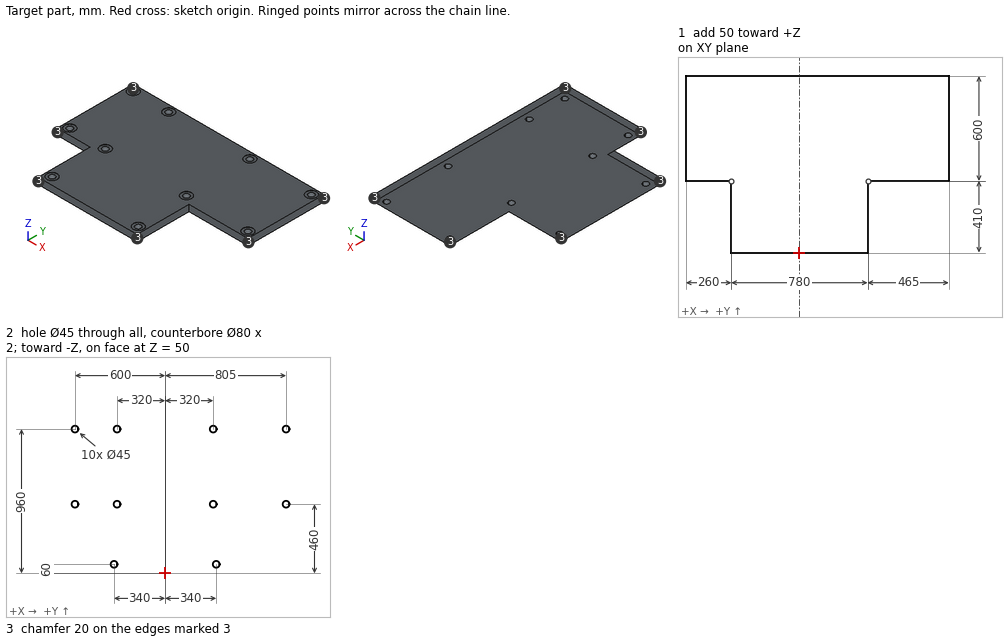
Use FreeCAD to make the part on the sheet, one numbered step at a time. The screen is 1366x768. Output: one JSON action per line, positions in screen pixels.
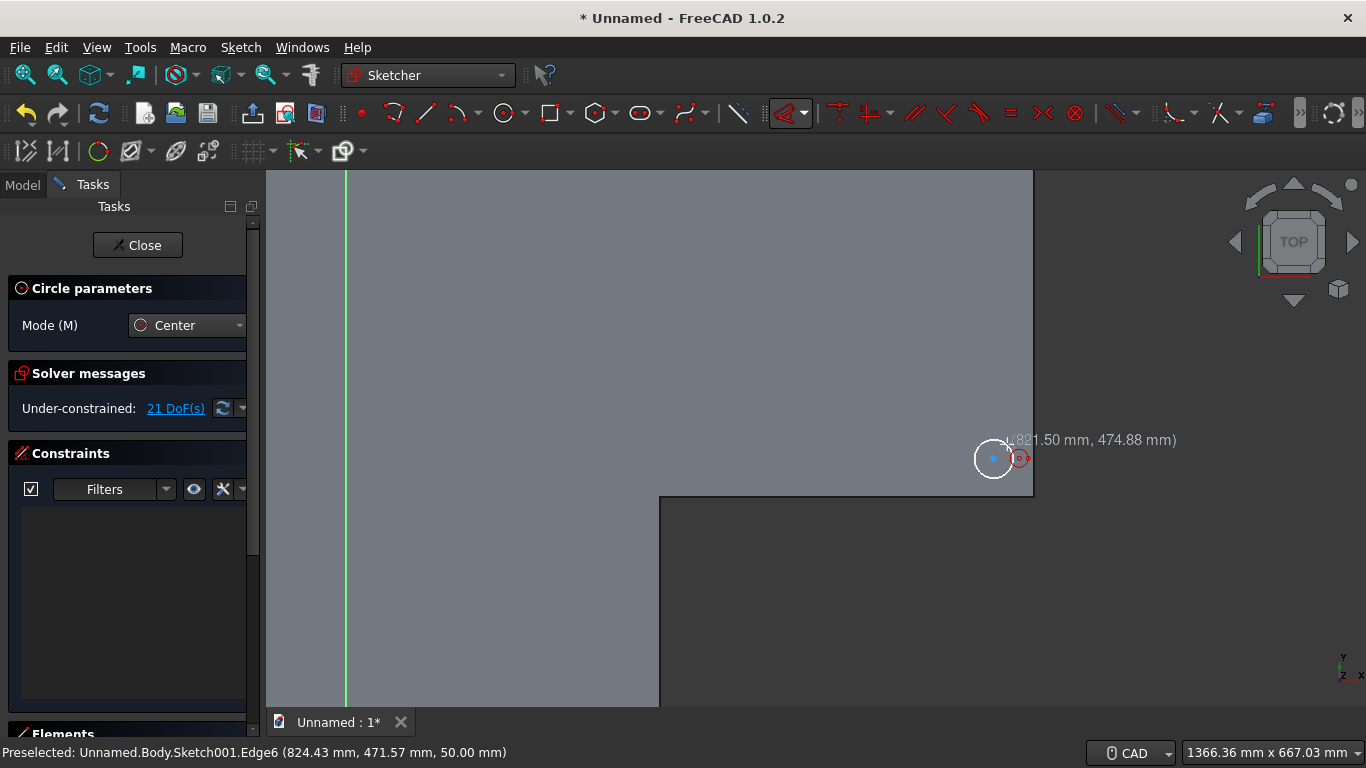
{"action": "scroll", "coordinate": [603, 457], "scroll_direction": "up", "scroll_amount": 2}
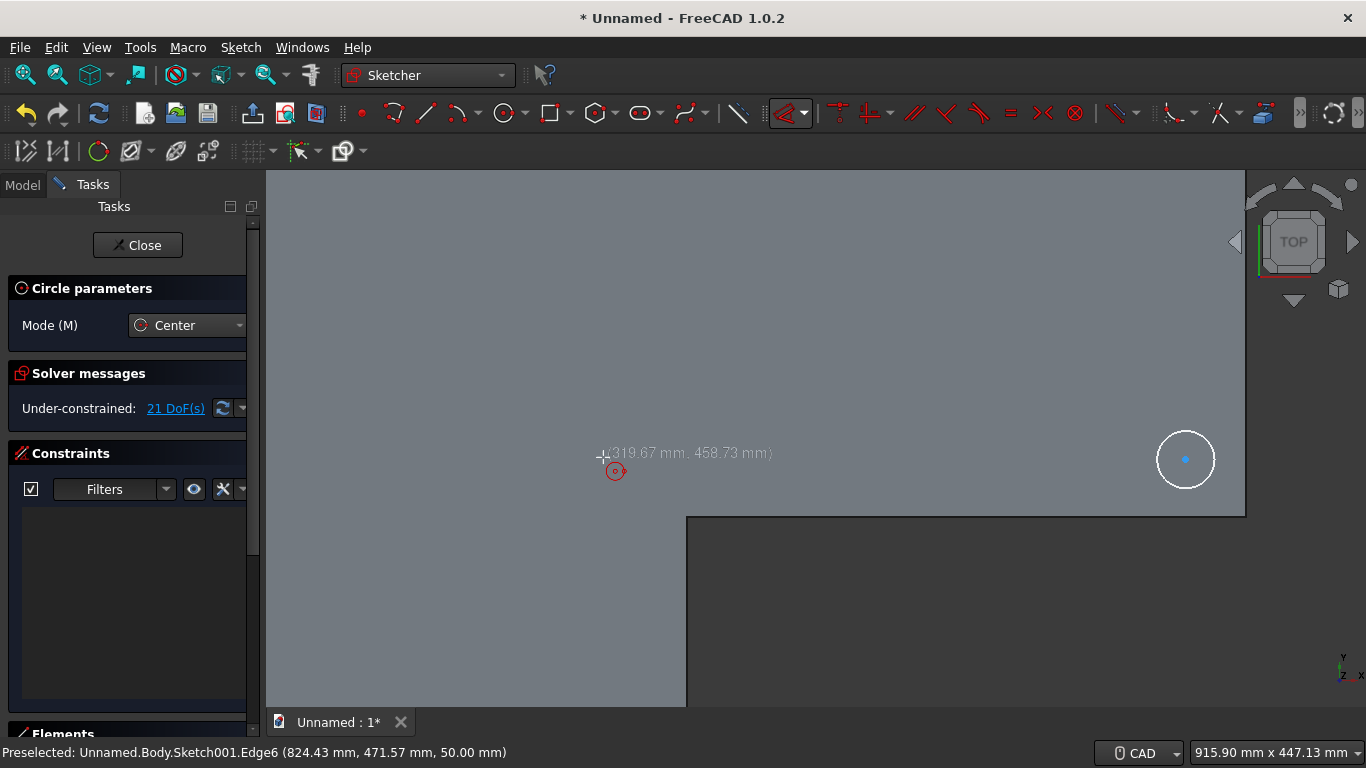
{"action": "scroll", "coordinate": [922, 447], "scroll_direction": "down", "scroll_amount": 6}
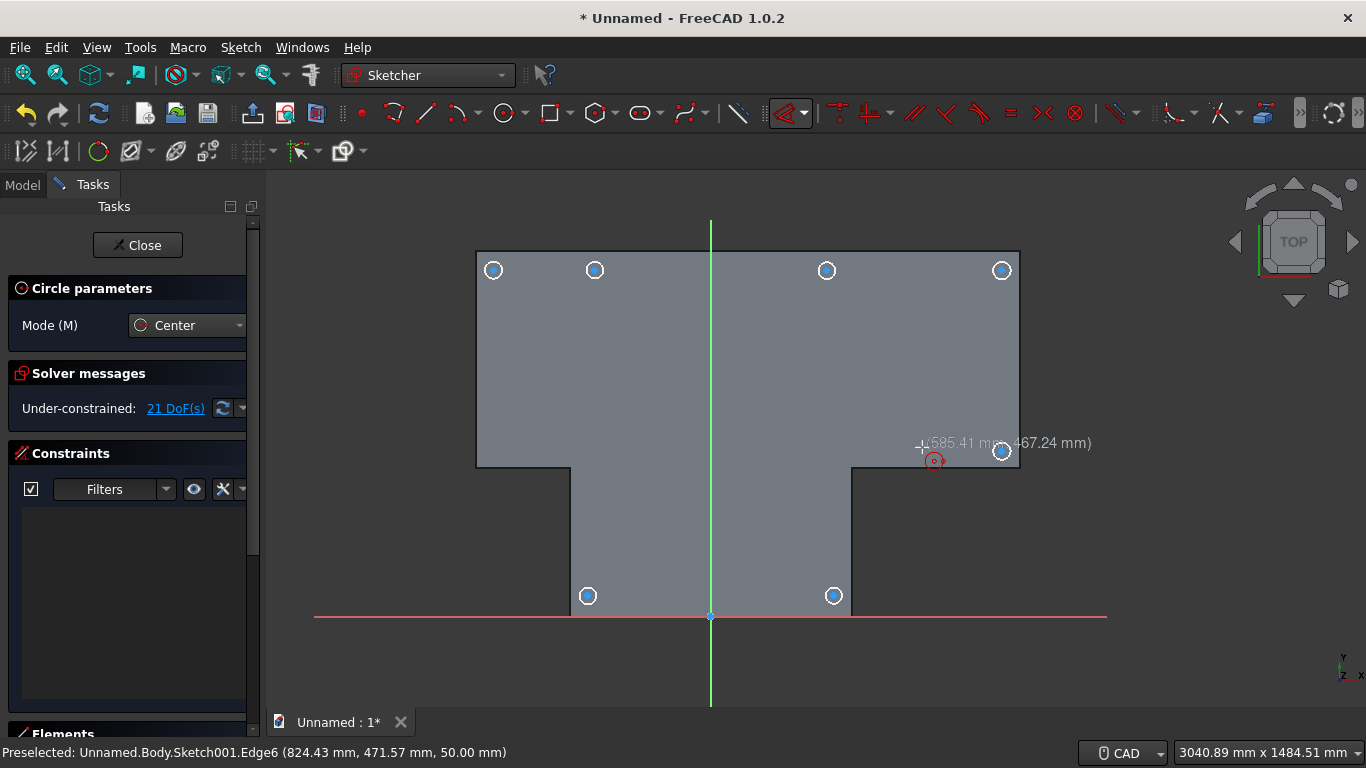
{"action": "left_click", "coordinate": [826, 450]}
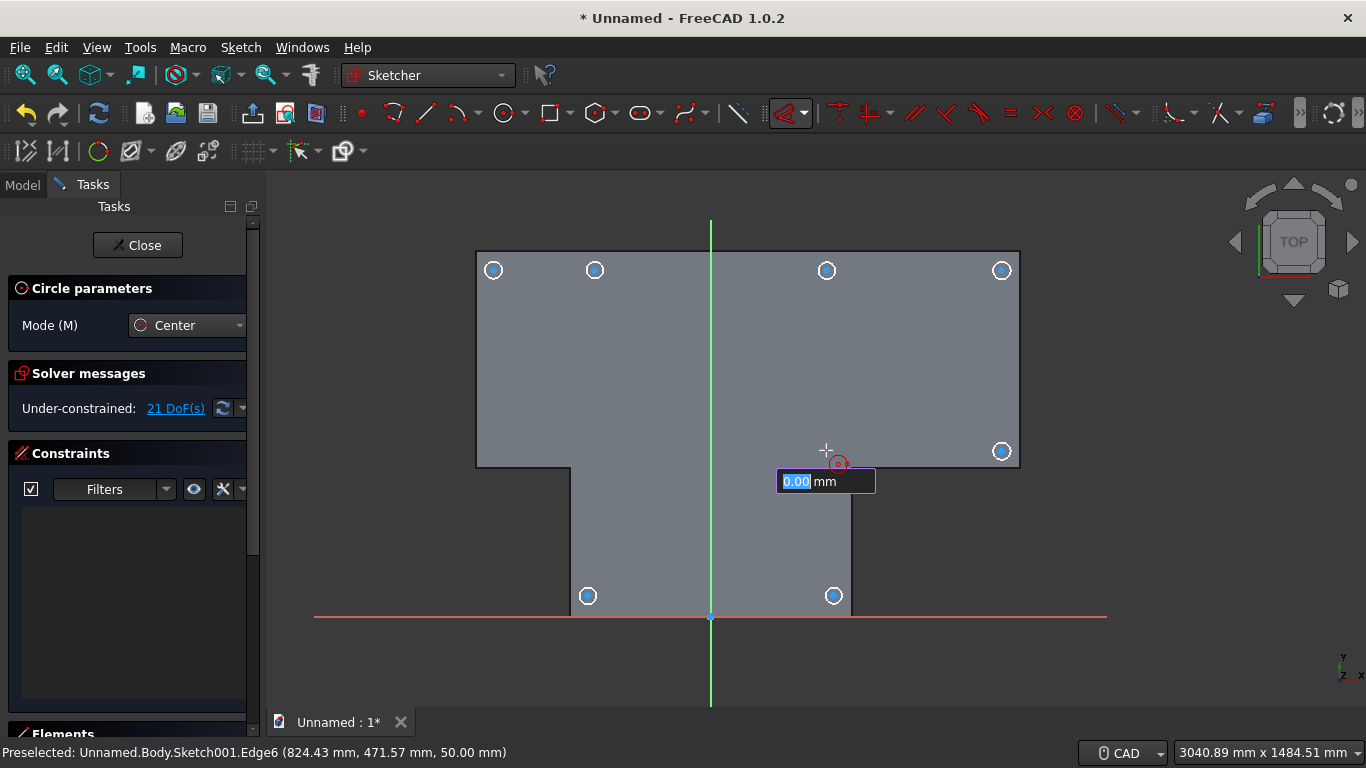
{"action": "scroll", "coordinate": [832, 445], "scroll_direction": "up", "scroll_amount": 4}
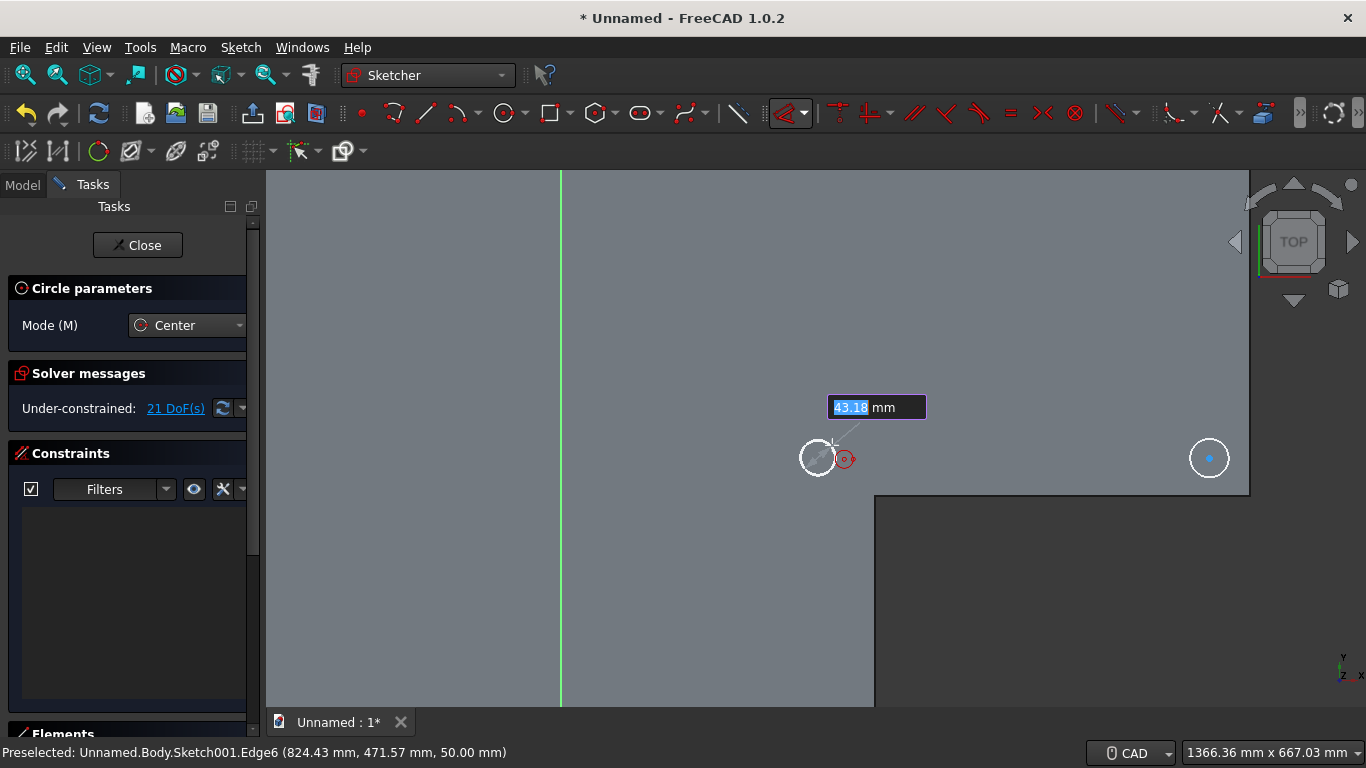
{"action": "left_click", "coordinate": [832, 443]}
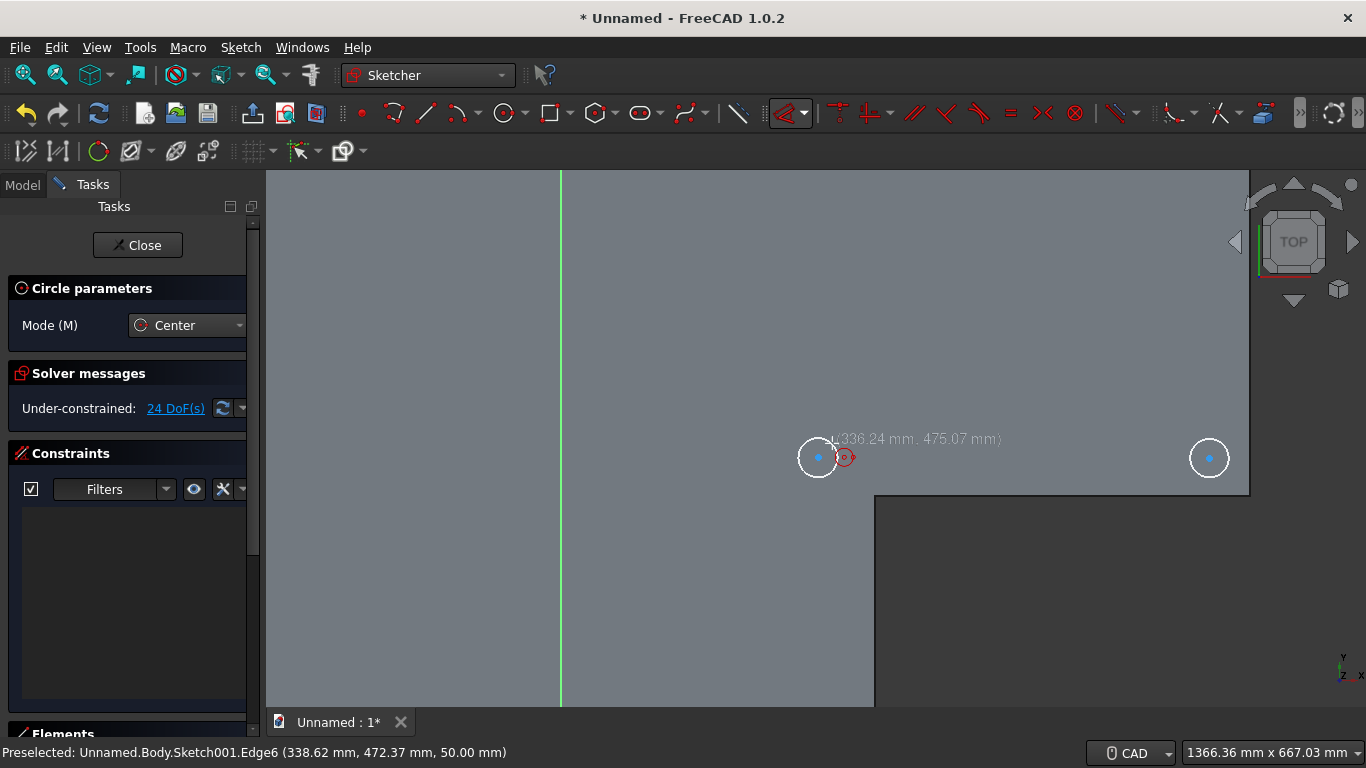
{"action": "scroll", "coordinate": [304, 456], "scroll_direction": "up", "scroll_amount": 2}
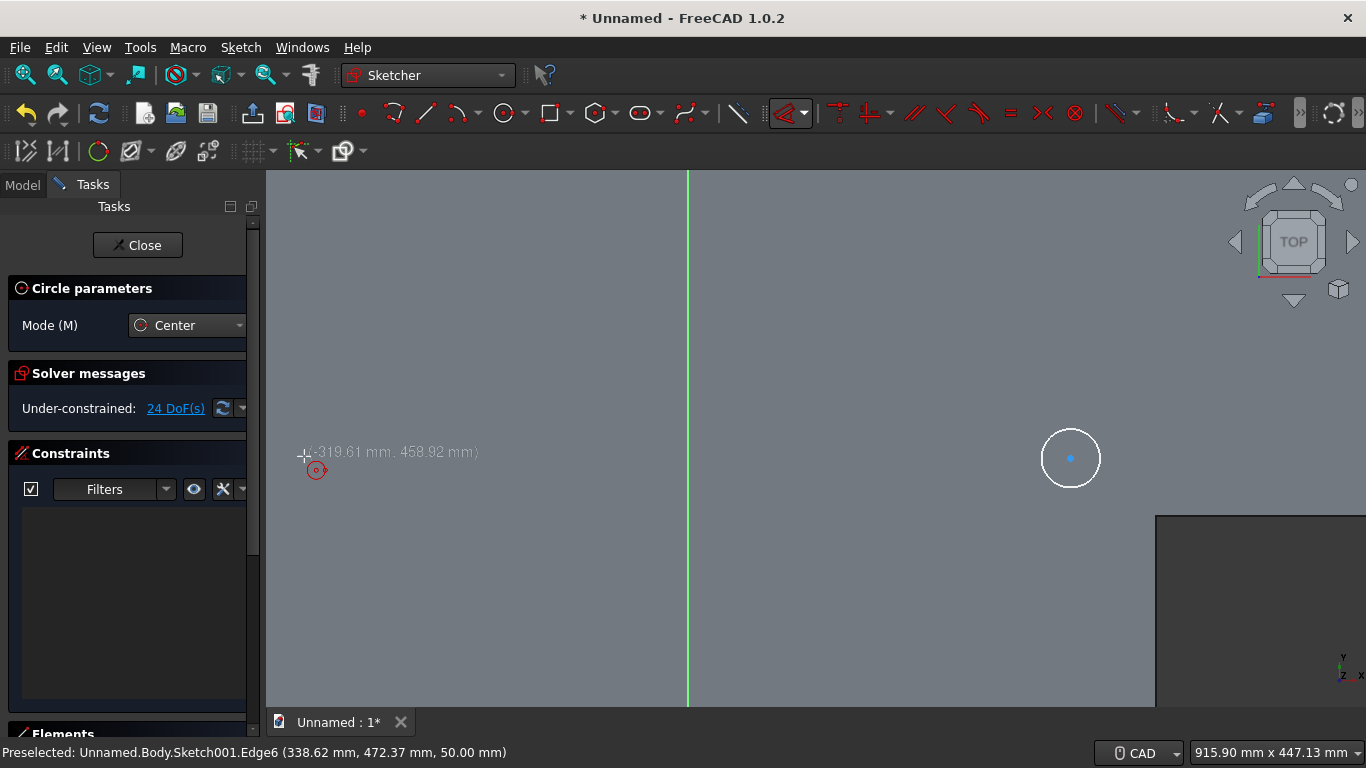
{"action": "scroll", "coordinate": [720, 447], "scroll_direction": "down", "scroll_amount": 6}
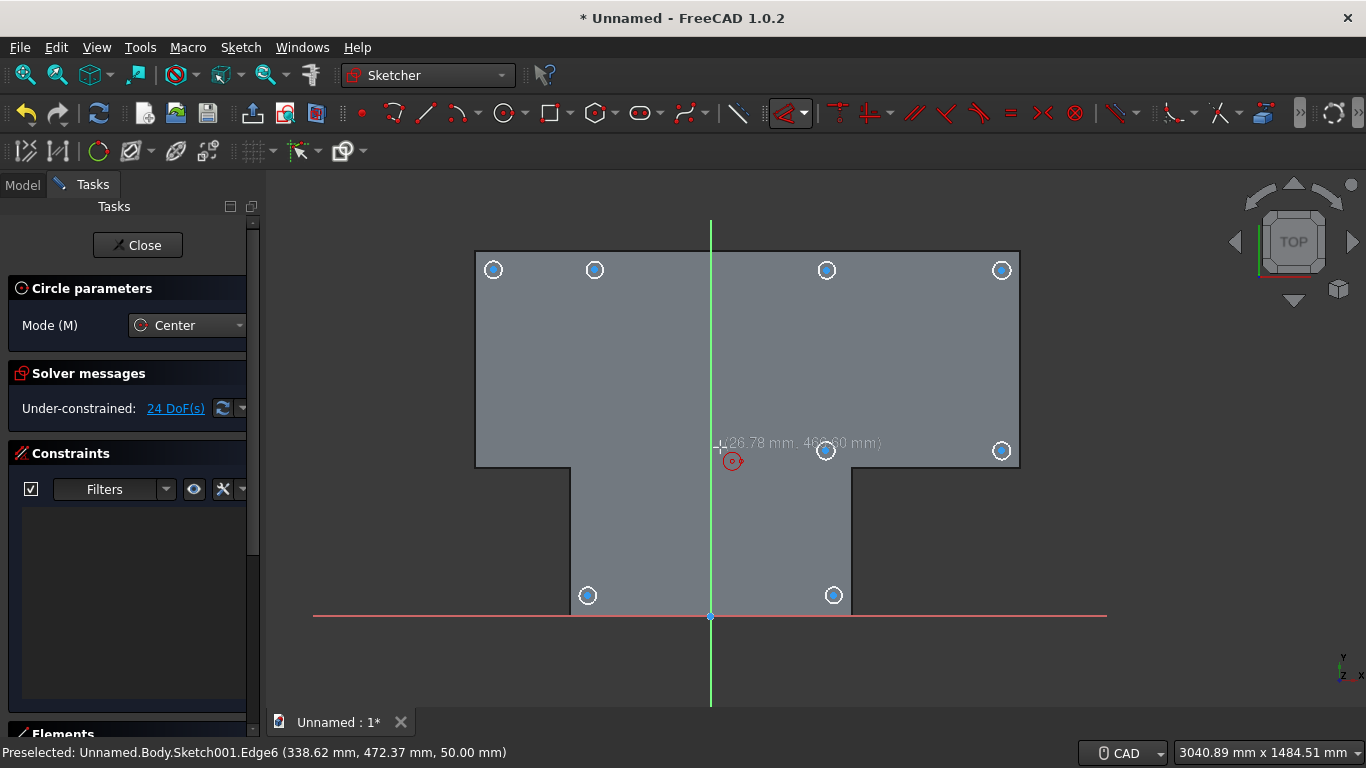
{"action": "left_click", "coordinate": [595, 450]}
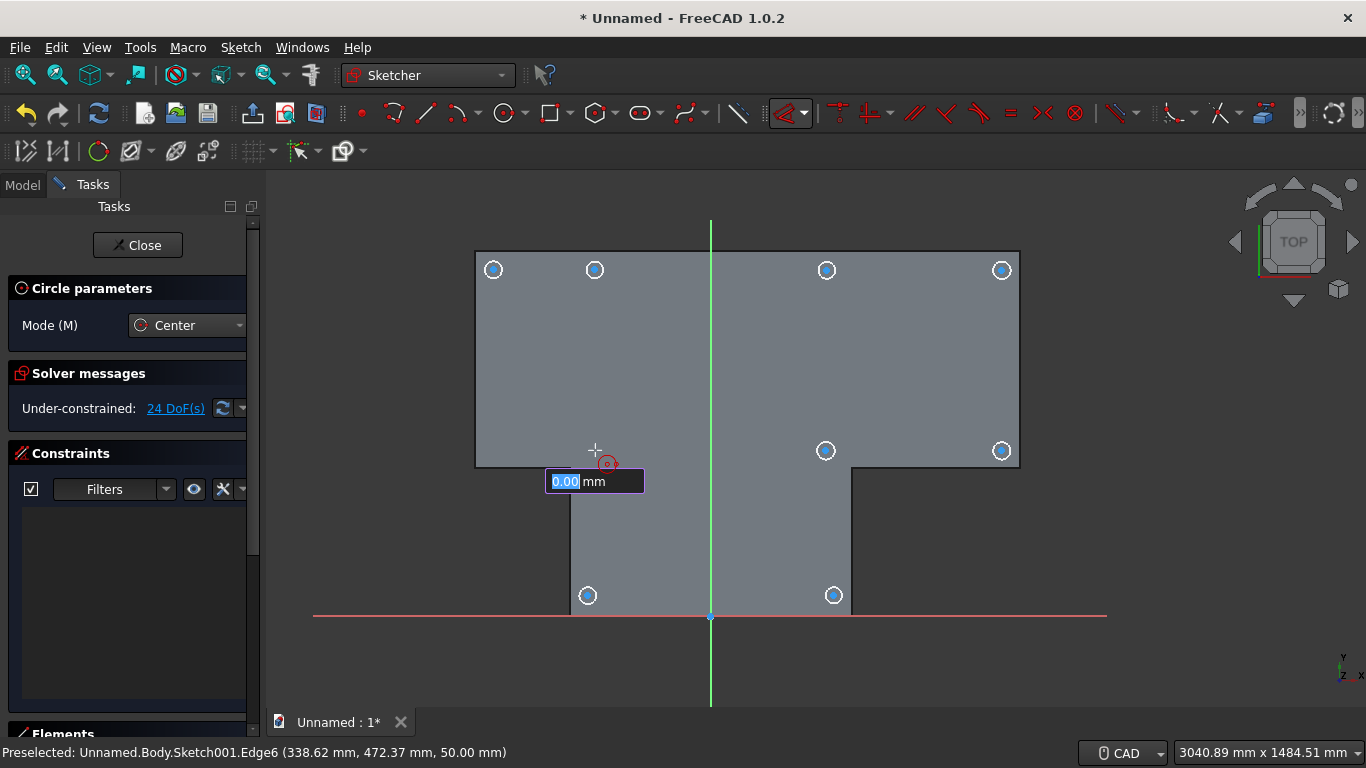
{"action": "scroll", "coordinate": [601, 444], "scroll_direction": "up", "scroll_amount": 4}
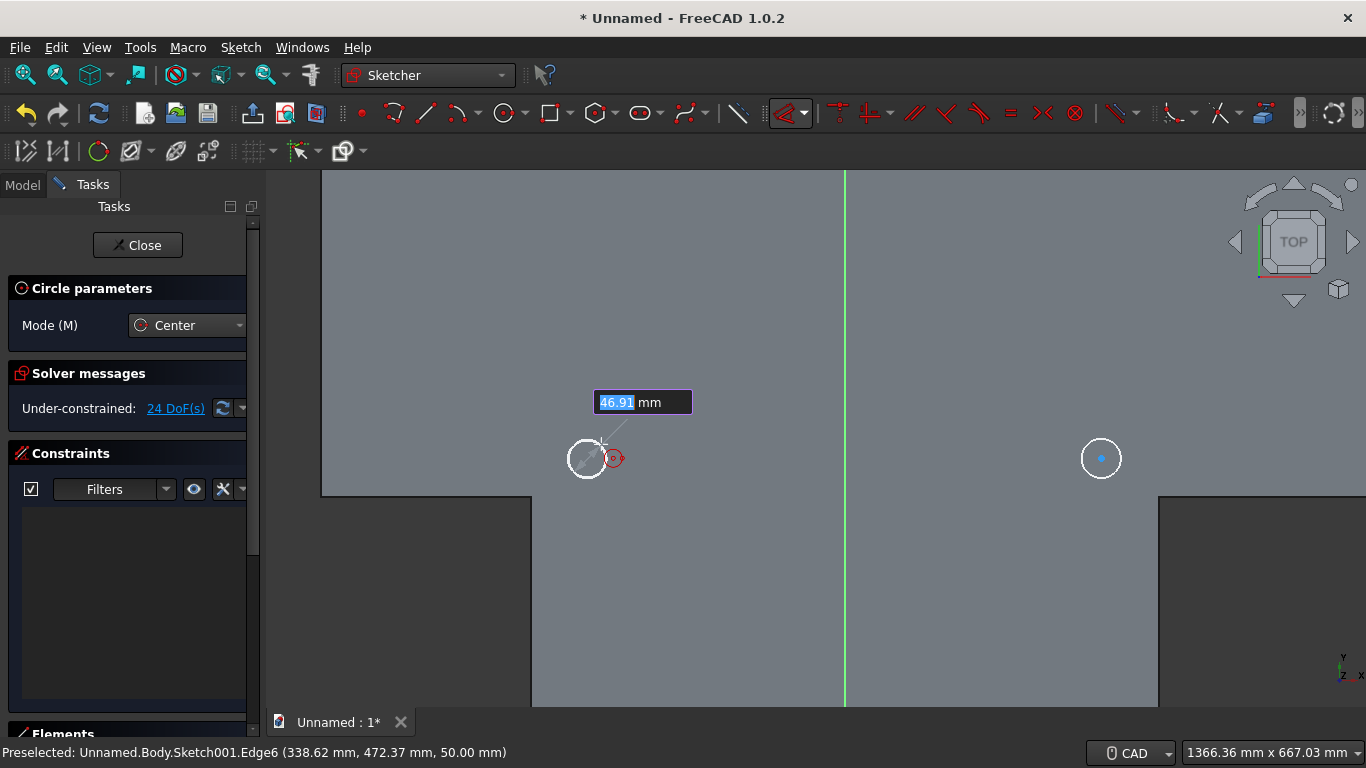
{"action": "left_click", "coordinate": [600, 444]}